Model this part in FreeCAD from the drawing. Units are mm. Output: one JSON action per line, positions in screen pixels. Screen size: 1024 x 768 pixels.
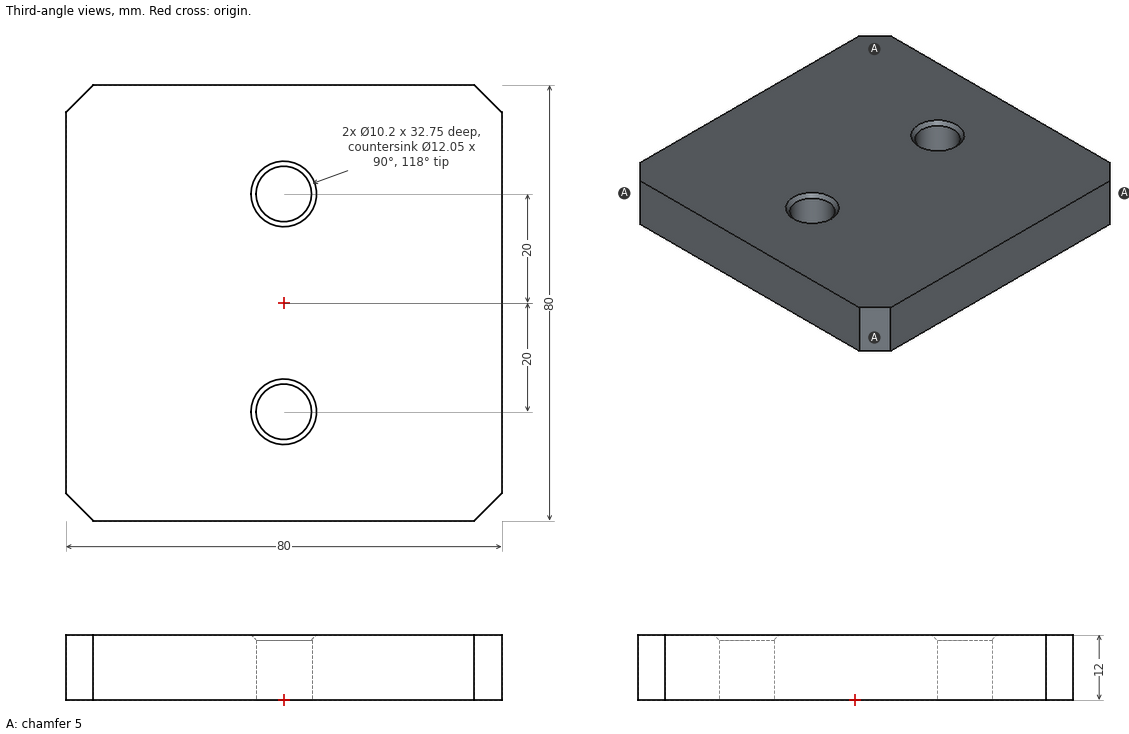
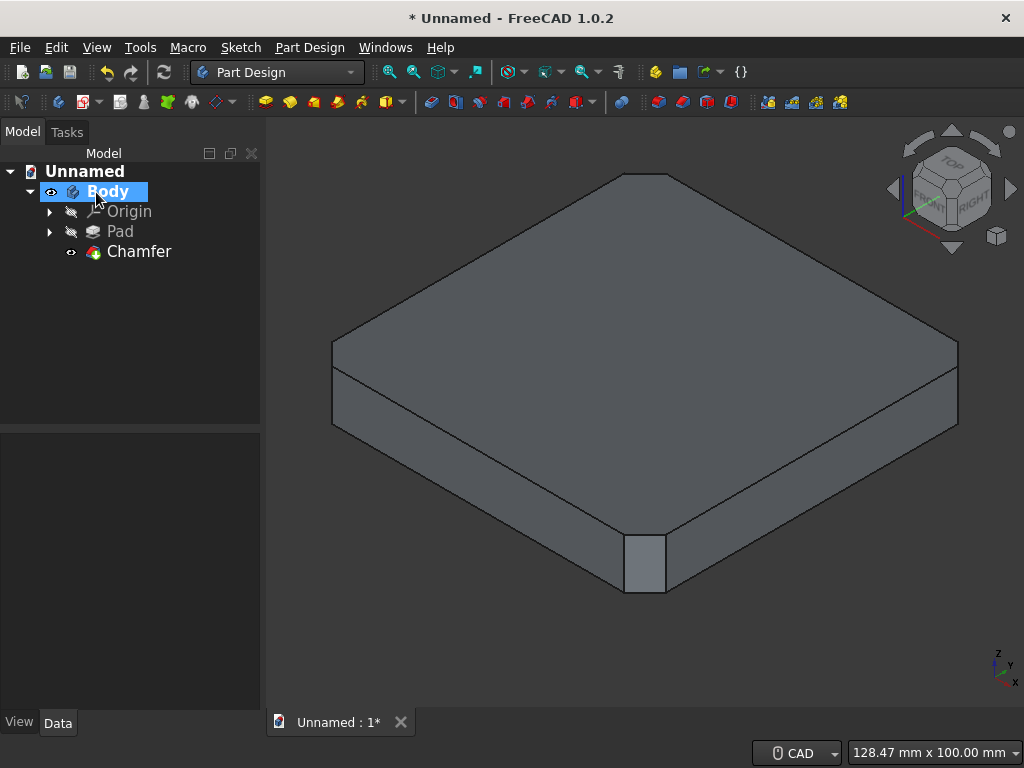
{"action": "left_click", "coordinate": [645, 353]}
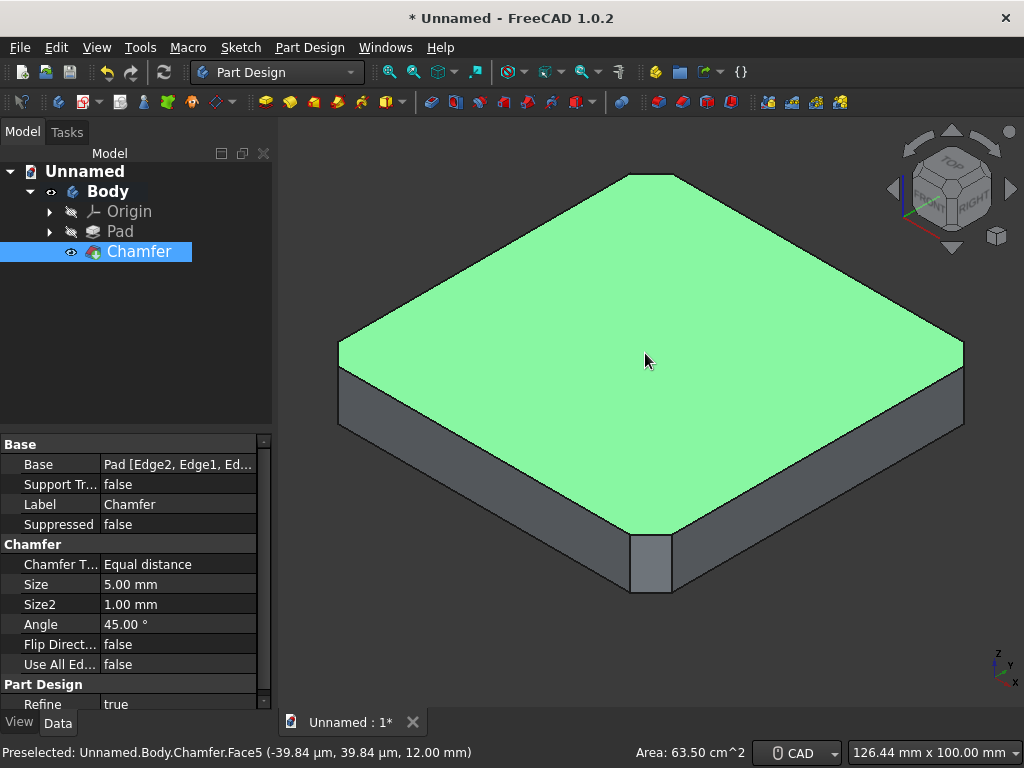
{"action": "left_click", "coordinate": [84, 102]}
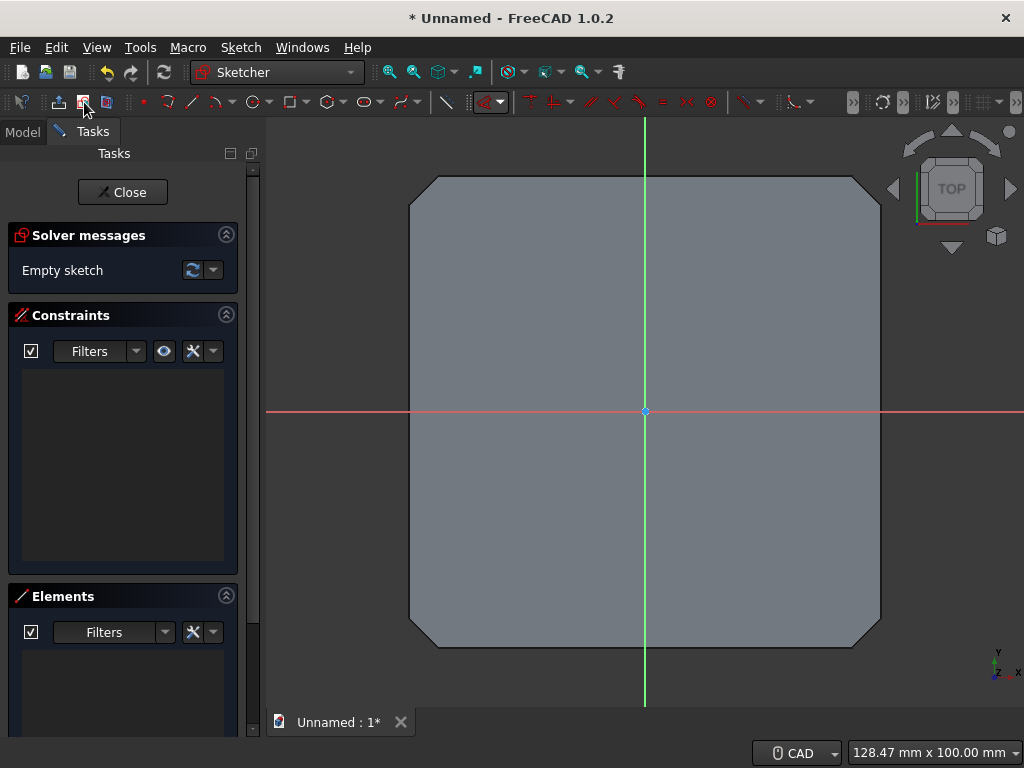
{"action": "left_click", "coordinate": [254, 102]}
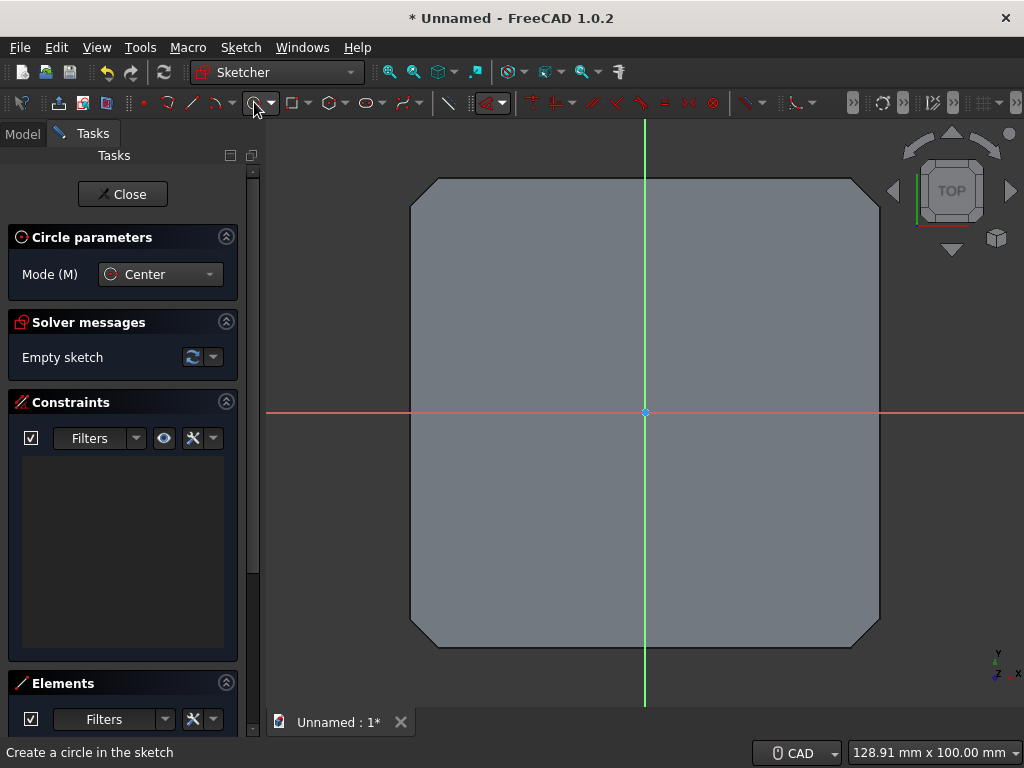
{"action": "left_click", "coordinate": [645, 295]}
{"action": "mouse_move", "coordinate": [666, 274]}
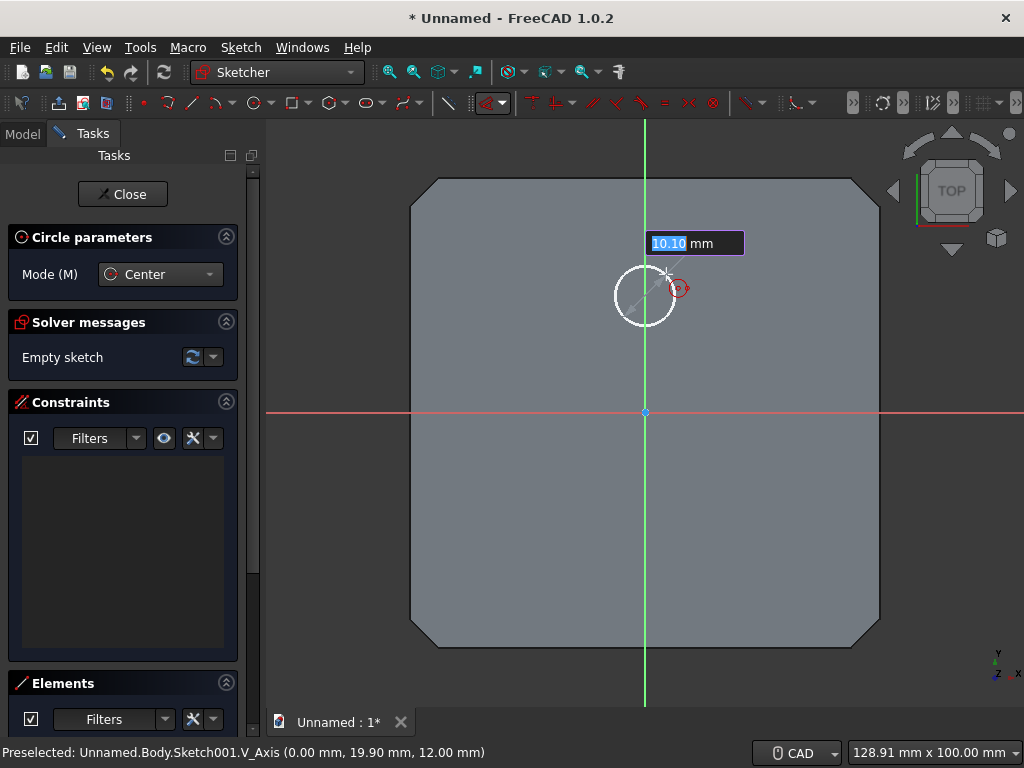
{"action": "type", "text": "10.2"}
{"action": "key", "text": "Return"}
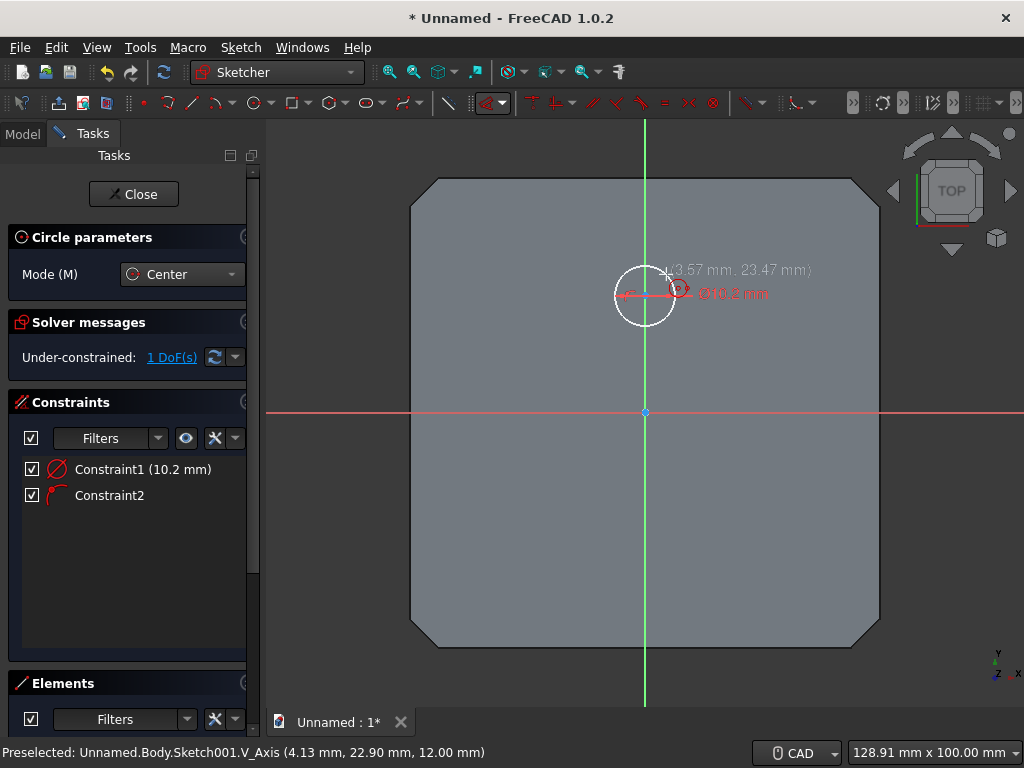
{"action": "left_click", "coordinate": [645, 531]}
{"action": "mouse_move", "coordinate": [666, 509]}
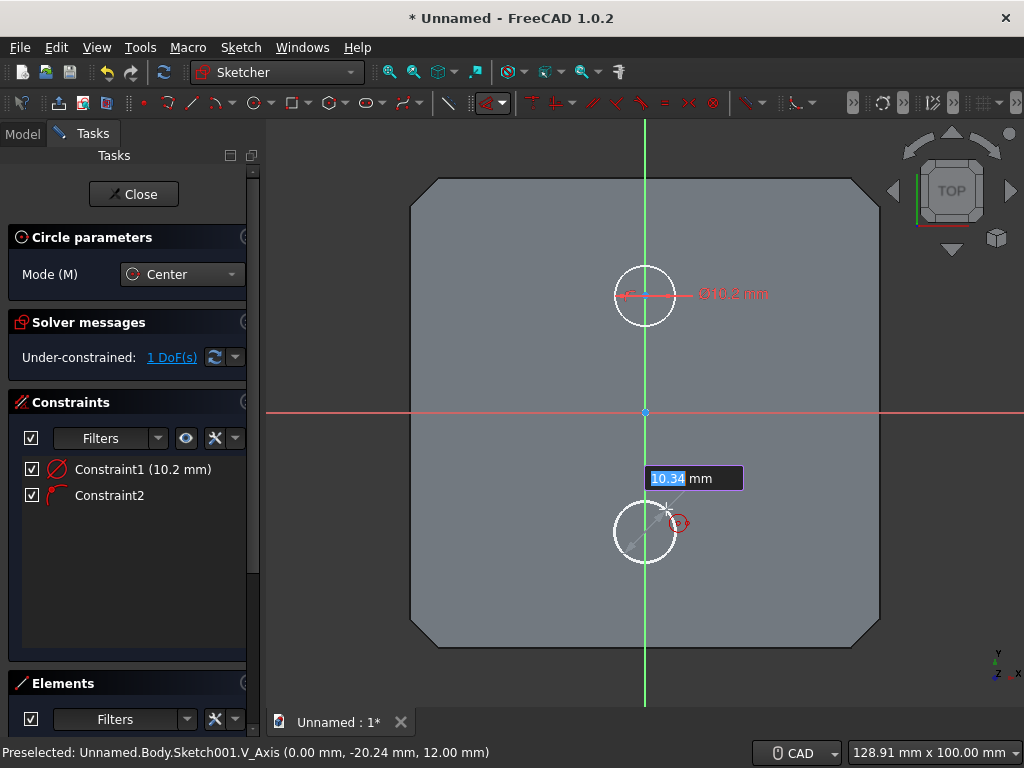
{"action": "type", "text": "10.2"}
{"action": "key", "text": "Return"}
{"action": "key", "text": "Escape"}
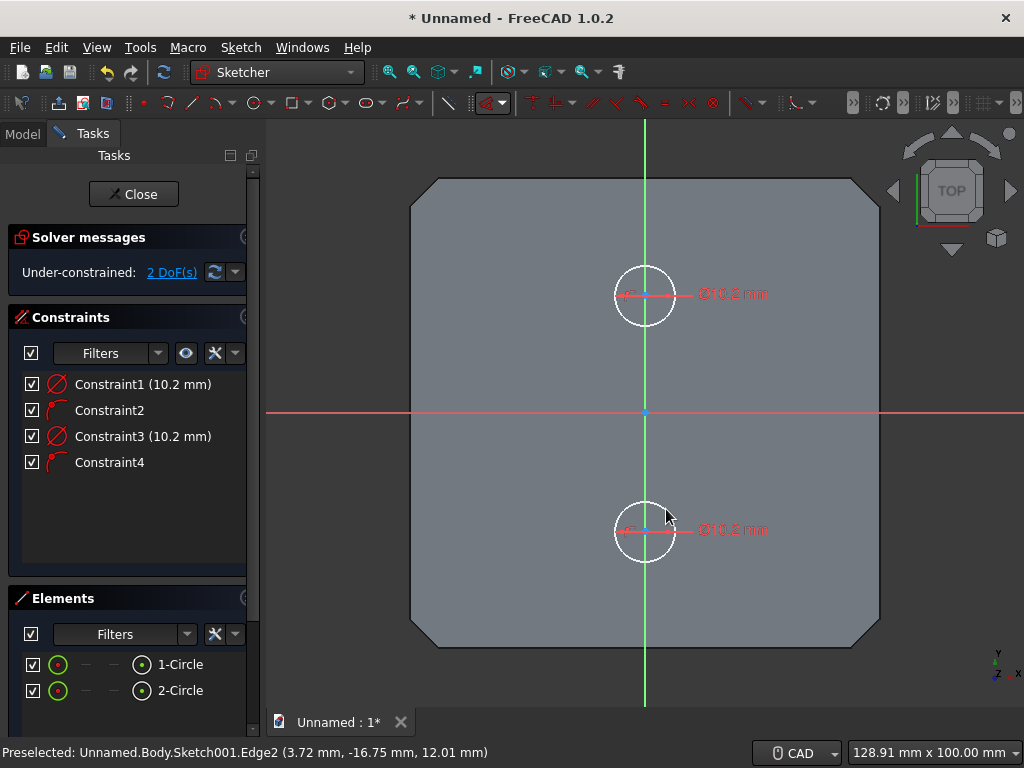
{"action": "left_click", "coordinate": [645, 296]}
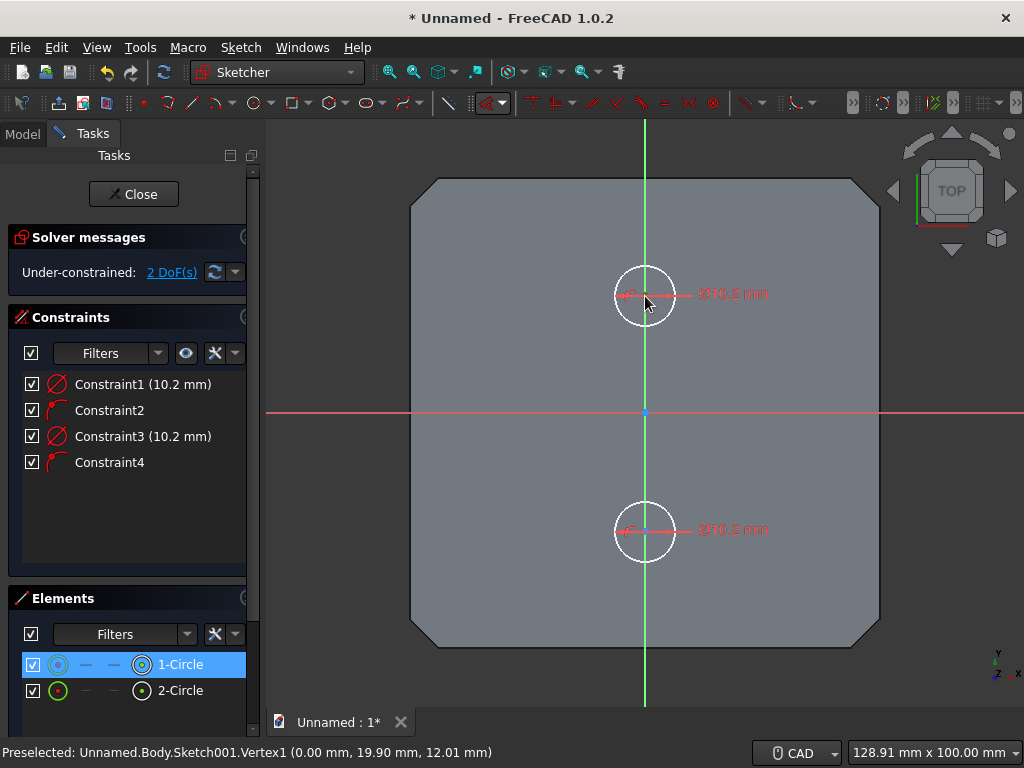
{"action": "left_click", "coordinate": [504, 104]}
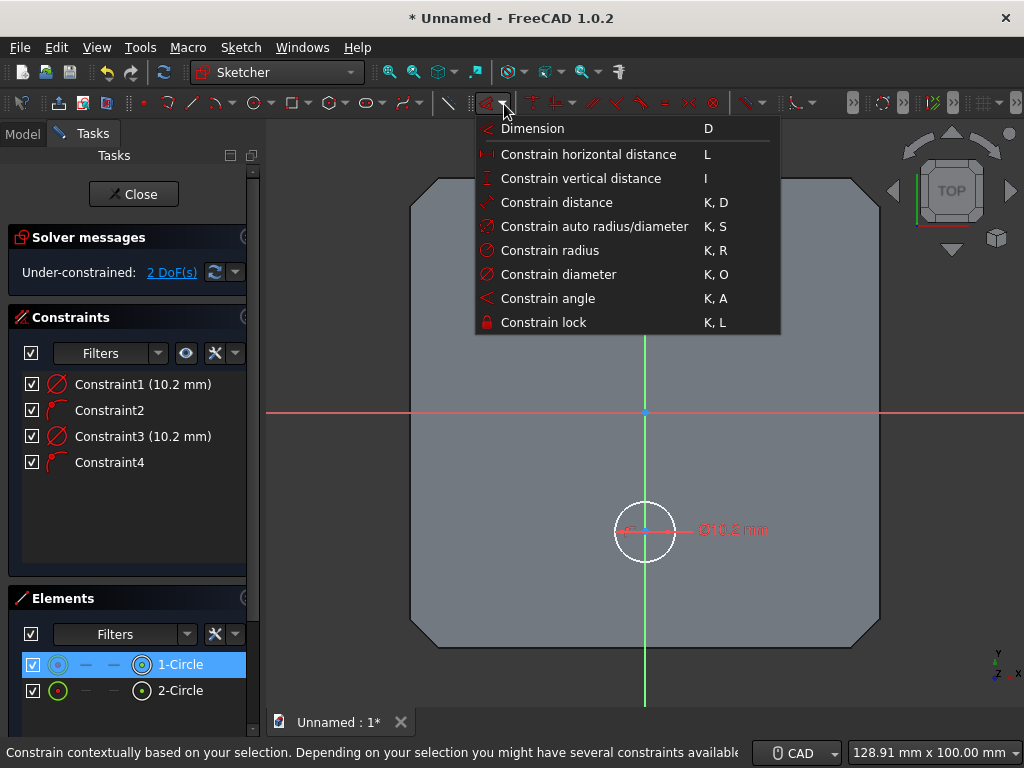
{"action": "left_click", "coordinate": [628, 178]}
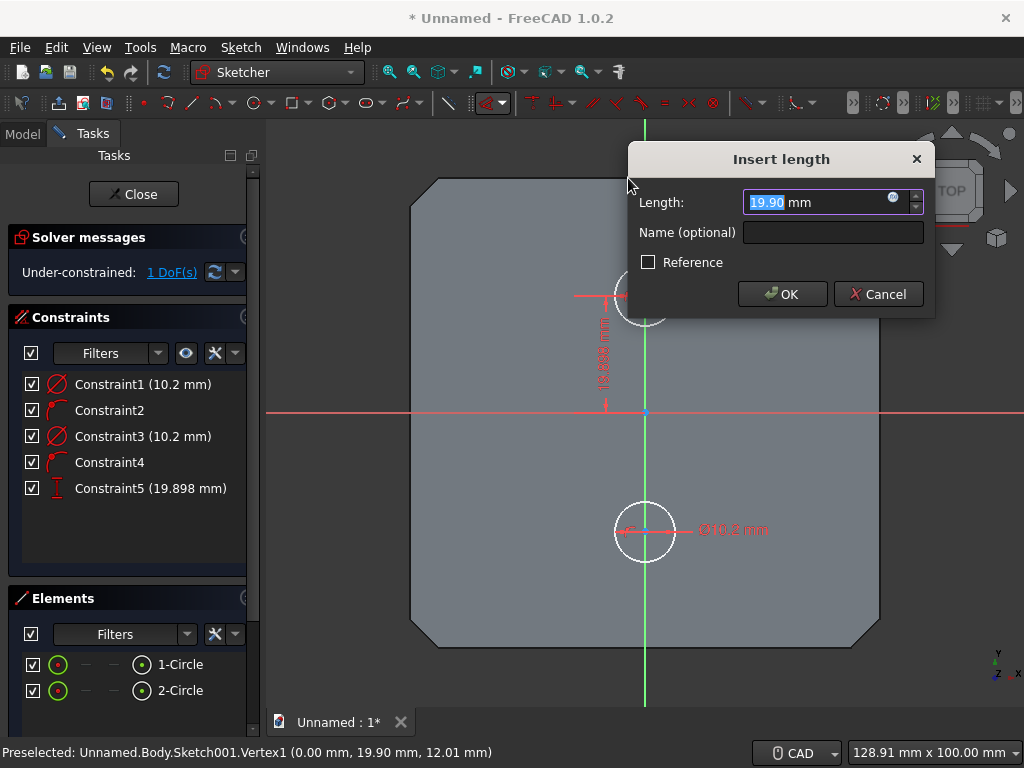
{"action": "type", "text": "20"}
{"action": "key", "text": "Return"}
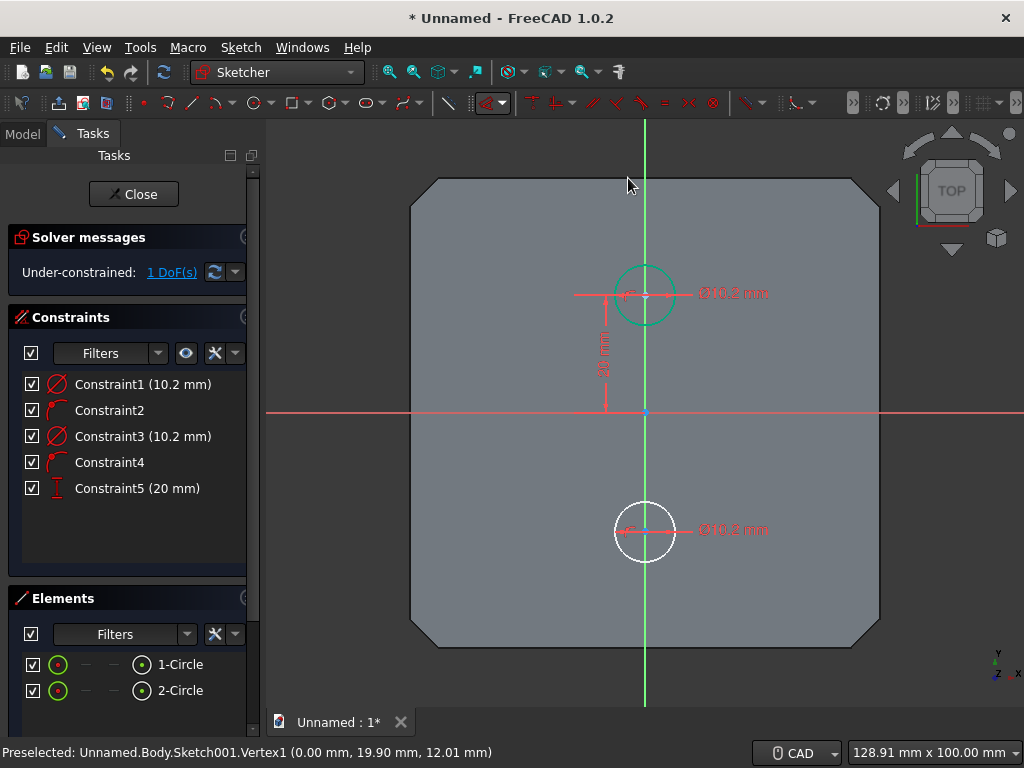
{"action": "left_click", "coordinate": [645, 532]}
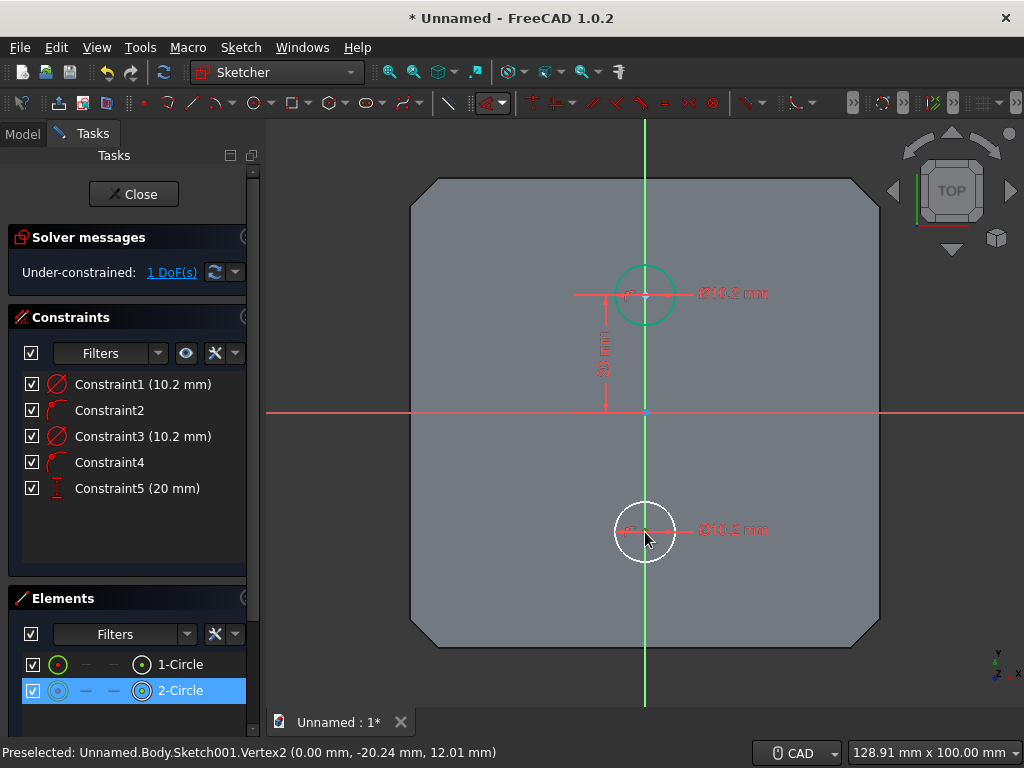
{"action": "key", "text": "i"}